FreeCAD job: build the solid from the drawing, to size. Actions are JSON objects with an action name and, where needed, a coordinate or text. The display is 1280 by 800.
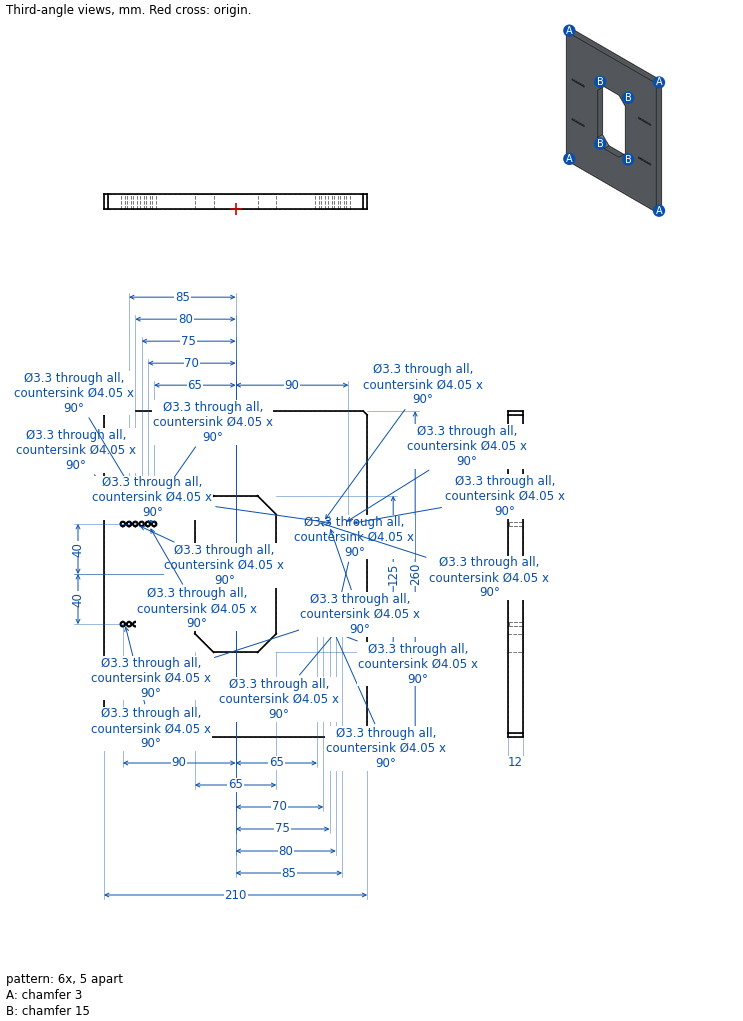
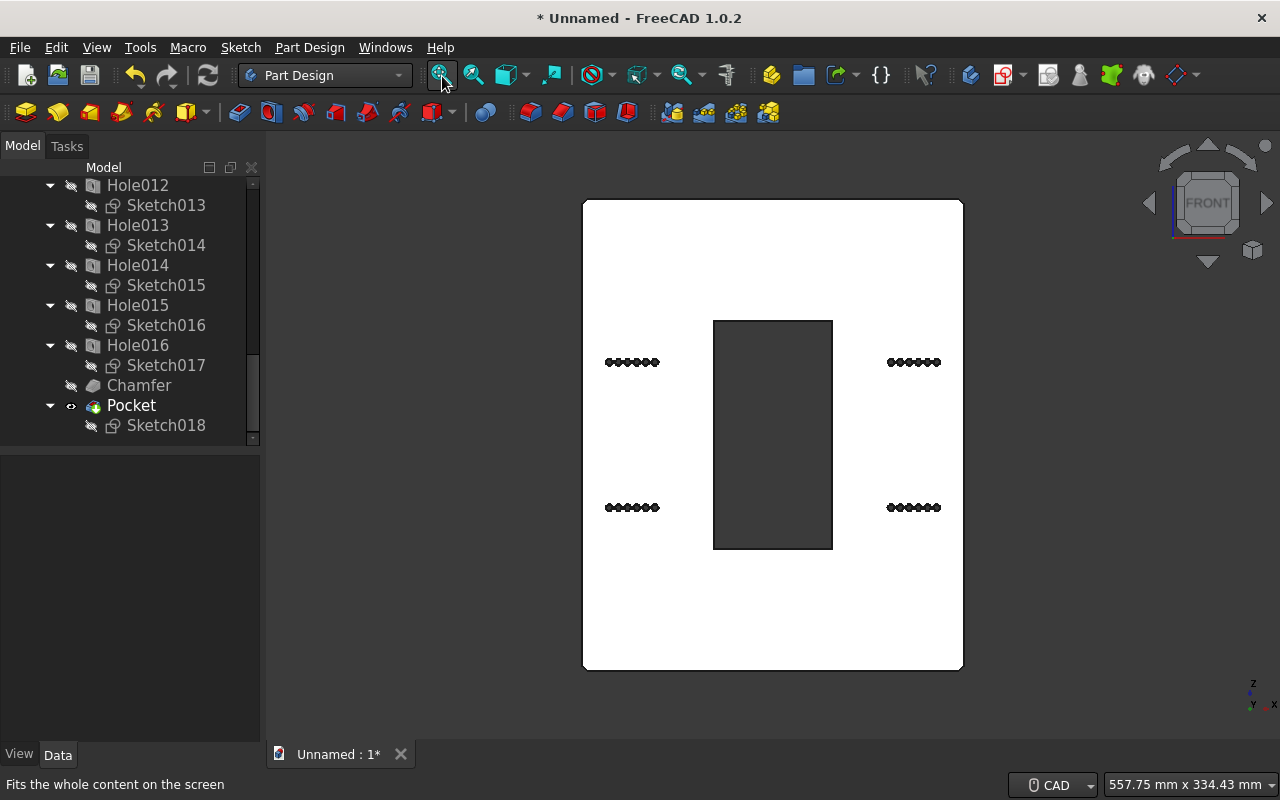
{"action": "scroll", "coordinate": [714, 548], "scroll_direction": "up", "scroll_amount": 4}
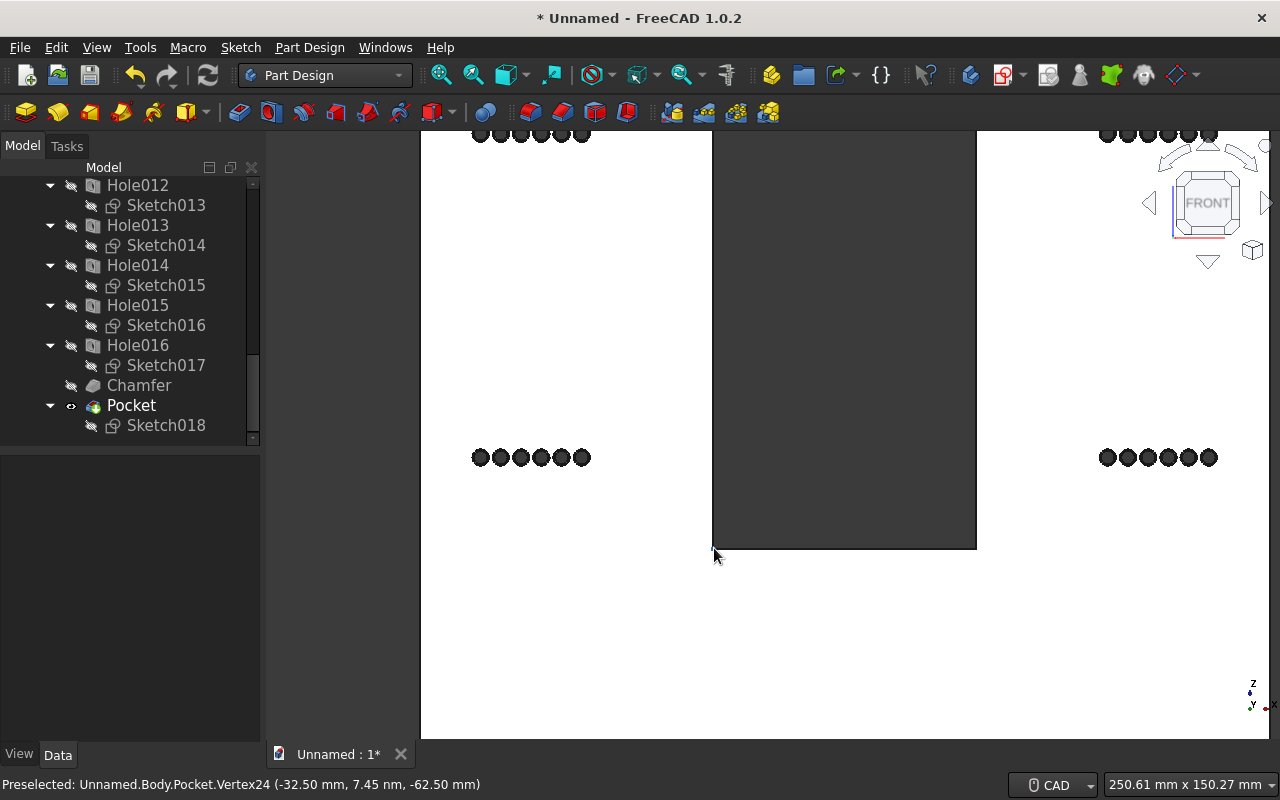
{"action": "left_click", "coordinate": [442, 76]}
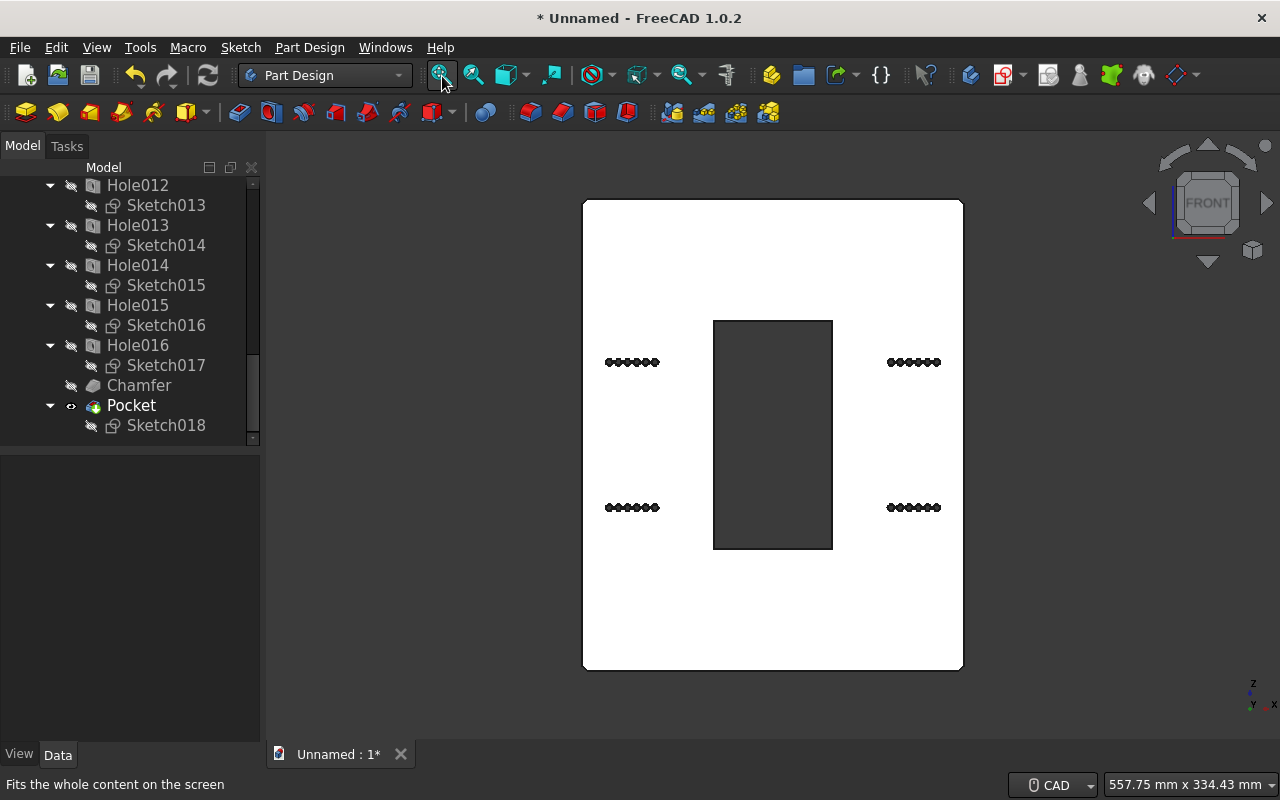
{"action": "key", "text": "3"}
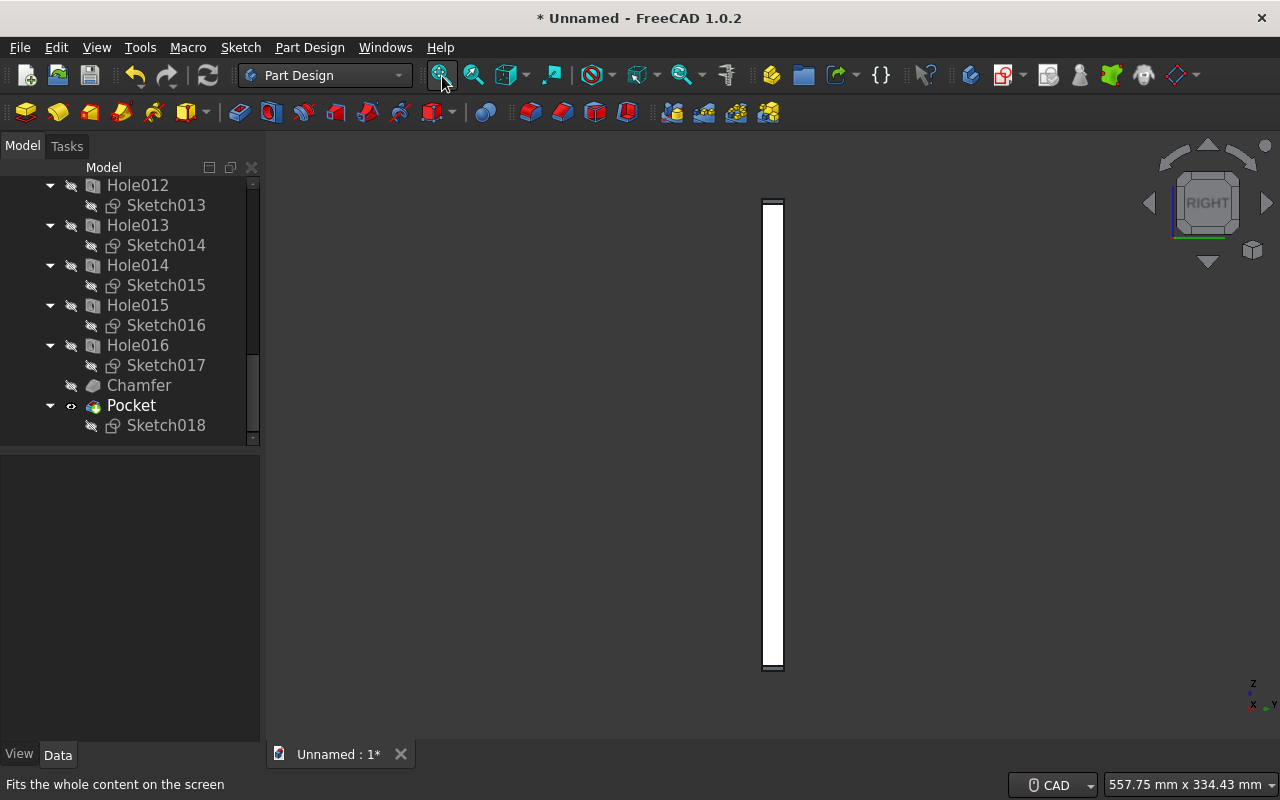
{"action": "scroll", "coordinate": [773, 548], "scroll_direction": "up", "scroll_amount": 4}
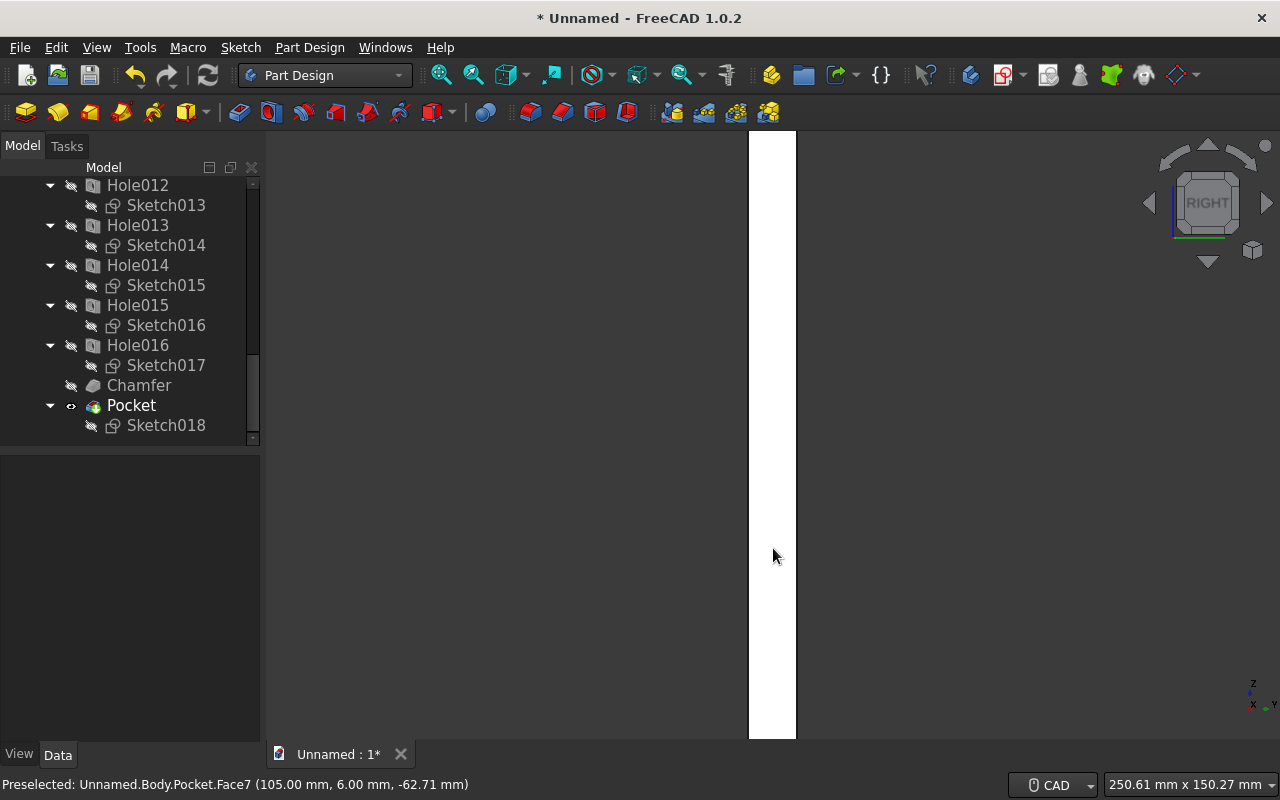
{"action": "left_click", "coordinate": [442, 76]}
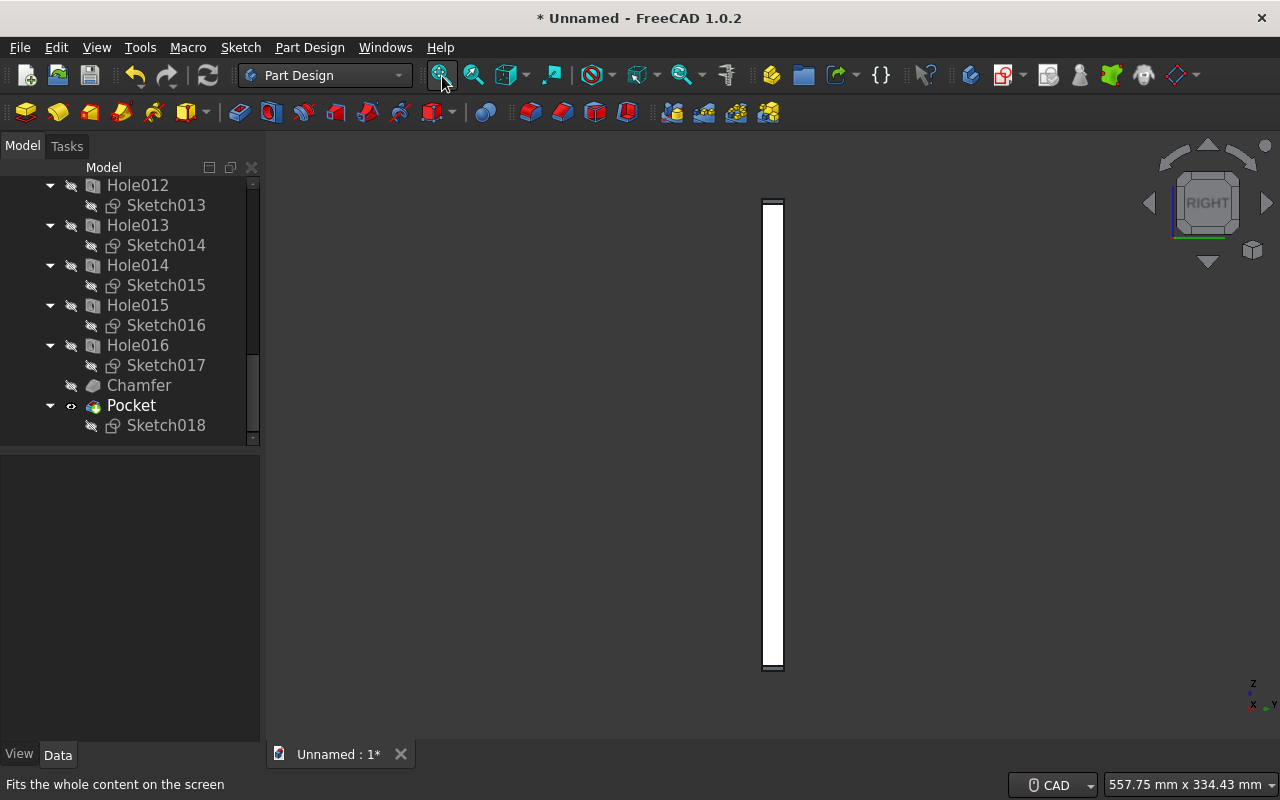
{"action": "key", "text": "5"}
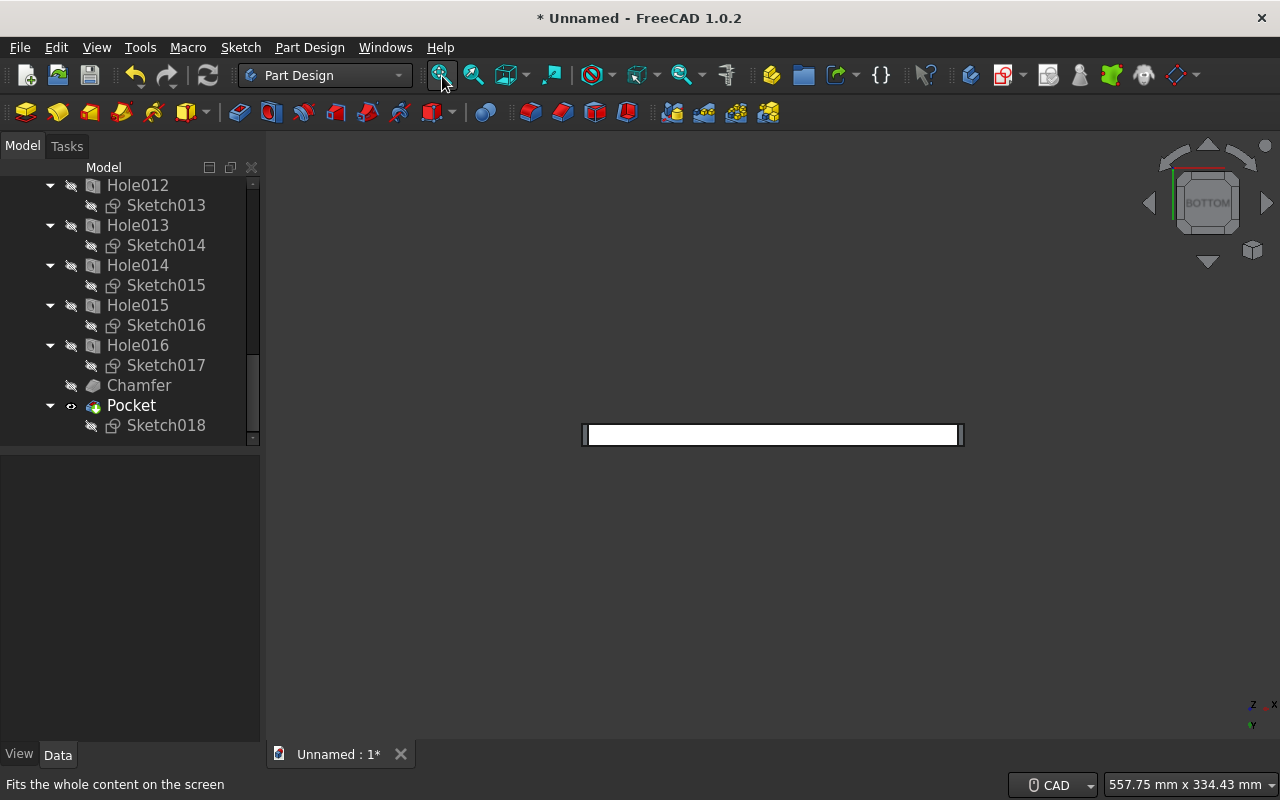
{"action": "left_click", "coordinate": [442, 76]}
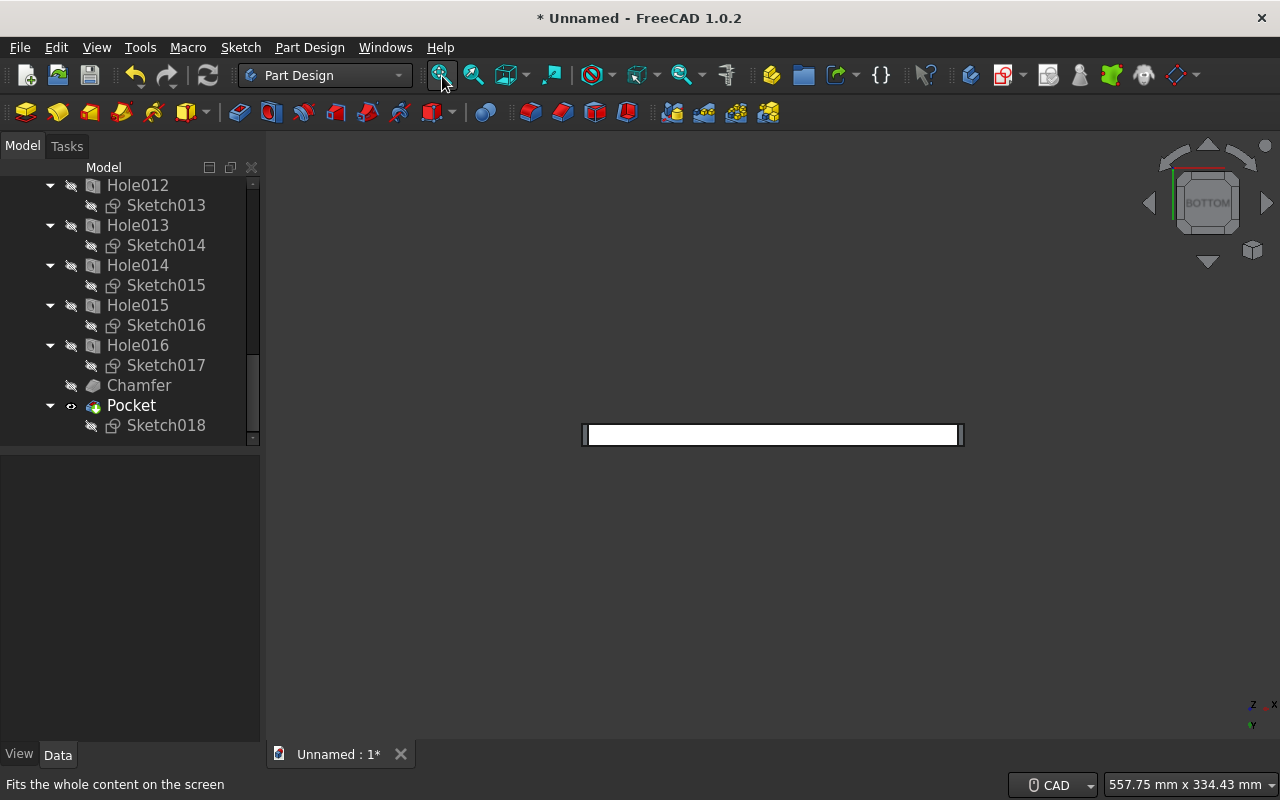
{"action": "scroll", "coordinate": [714, 434], "scroll_direction": "up", "scroll_amount": 4}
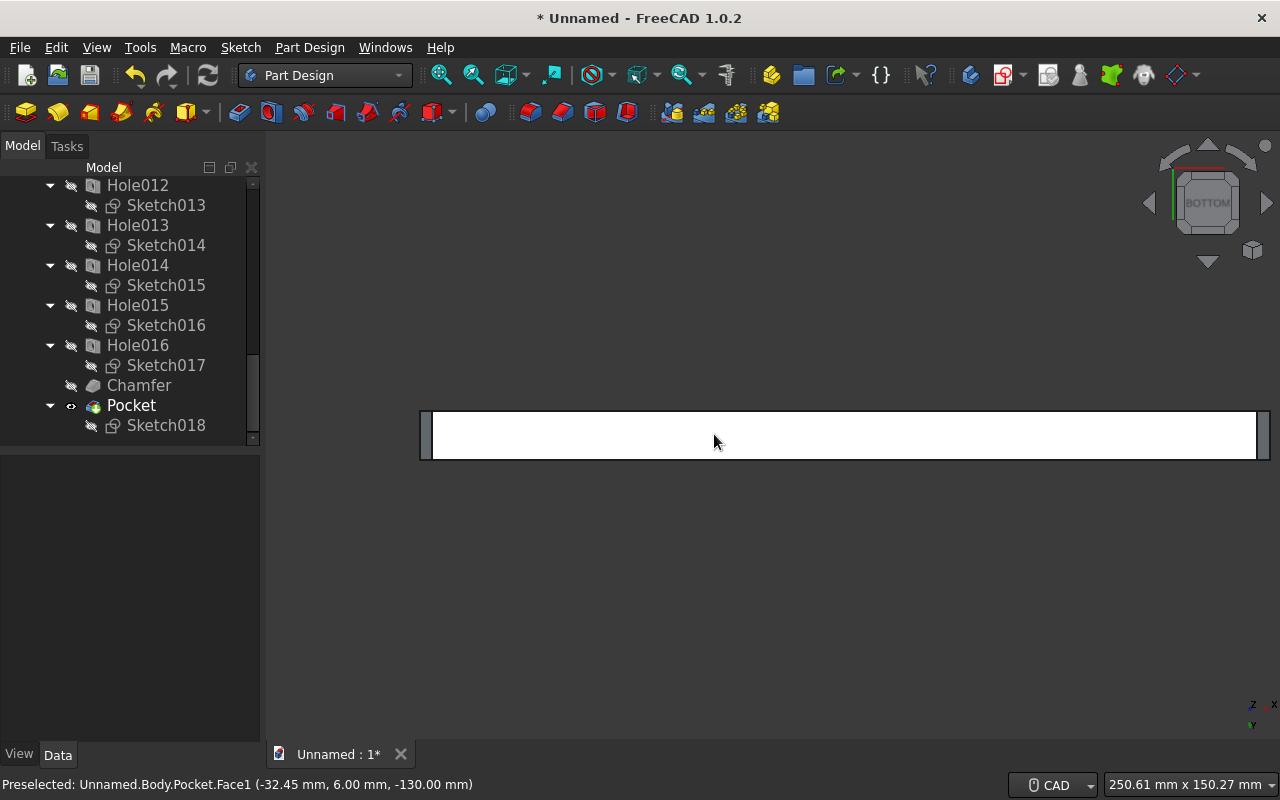
{"action": "left_click", "coordinate": [442, 76]}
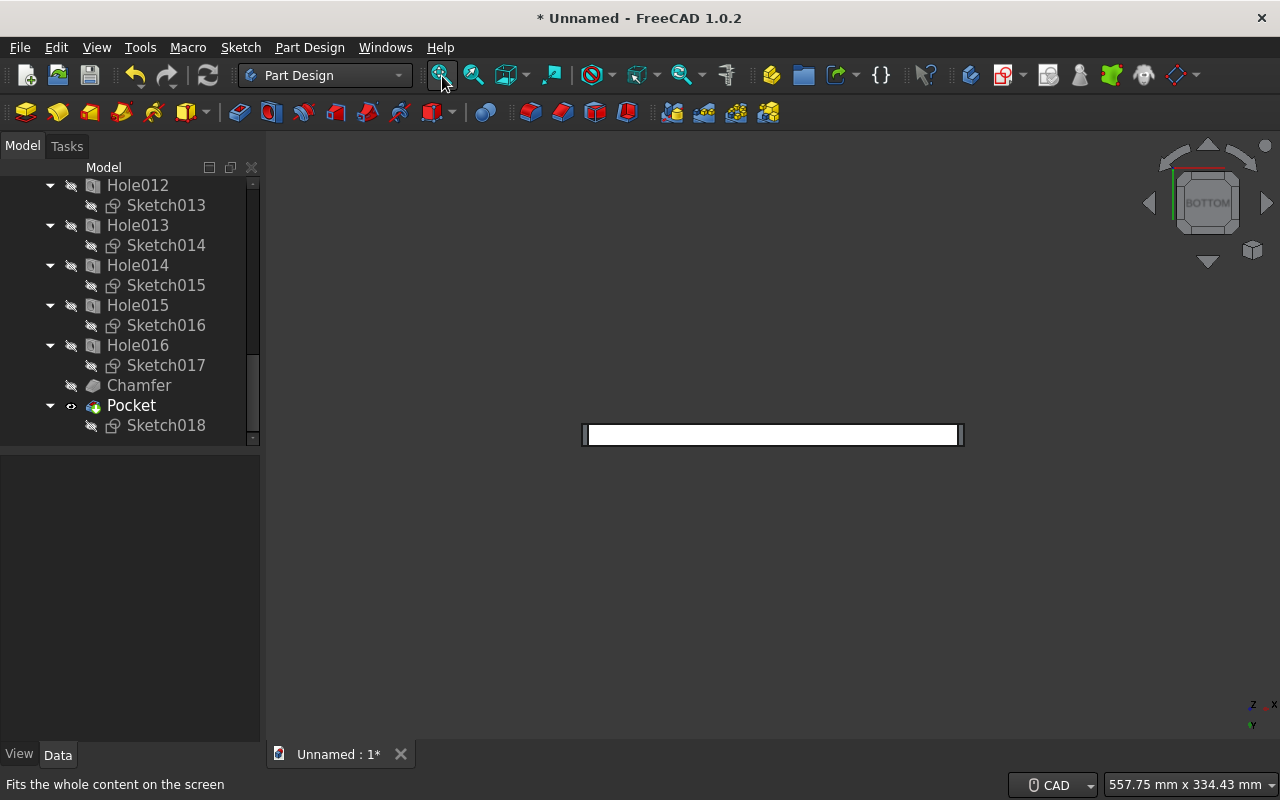
{"action": "key", "text": "4"}